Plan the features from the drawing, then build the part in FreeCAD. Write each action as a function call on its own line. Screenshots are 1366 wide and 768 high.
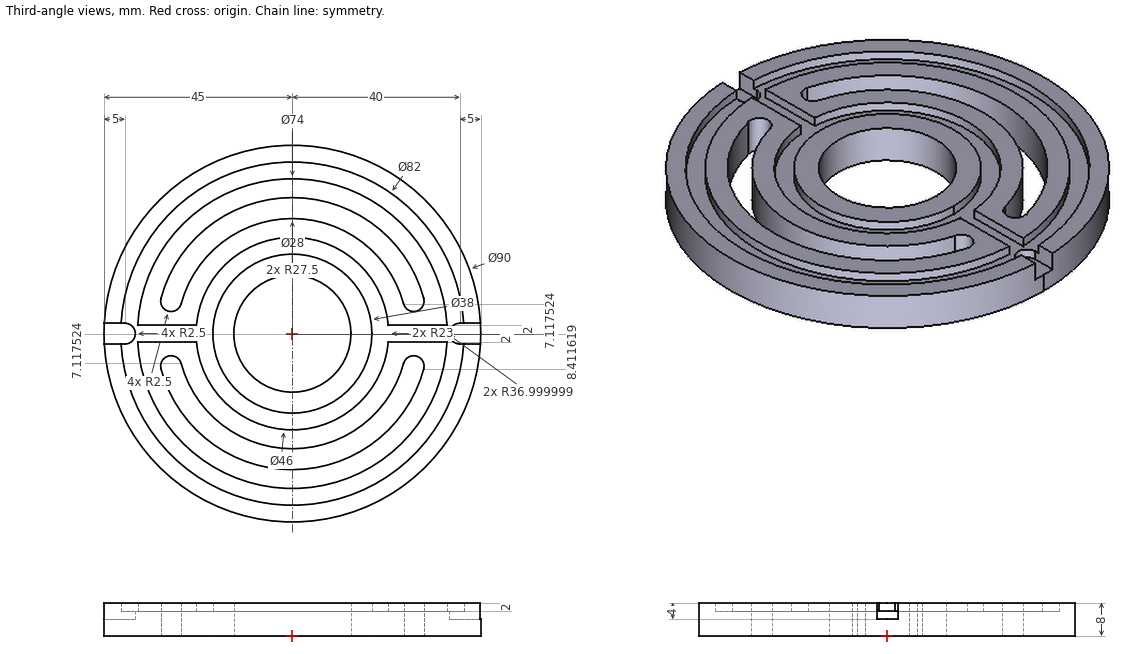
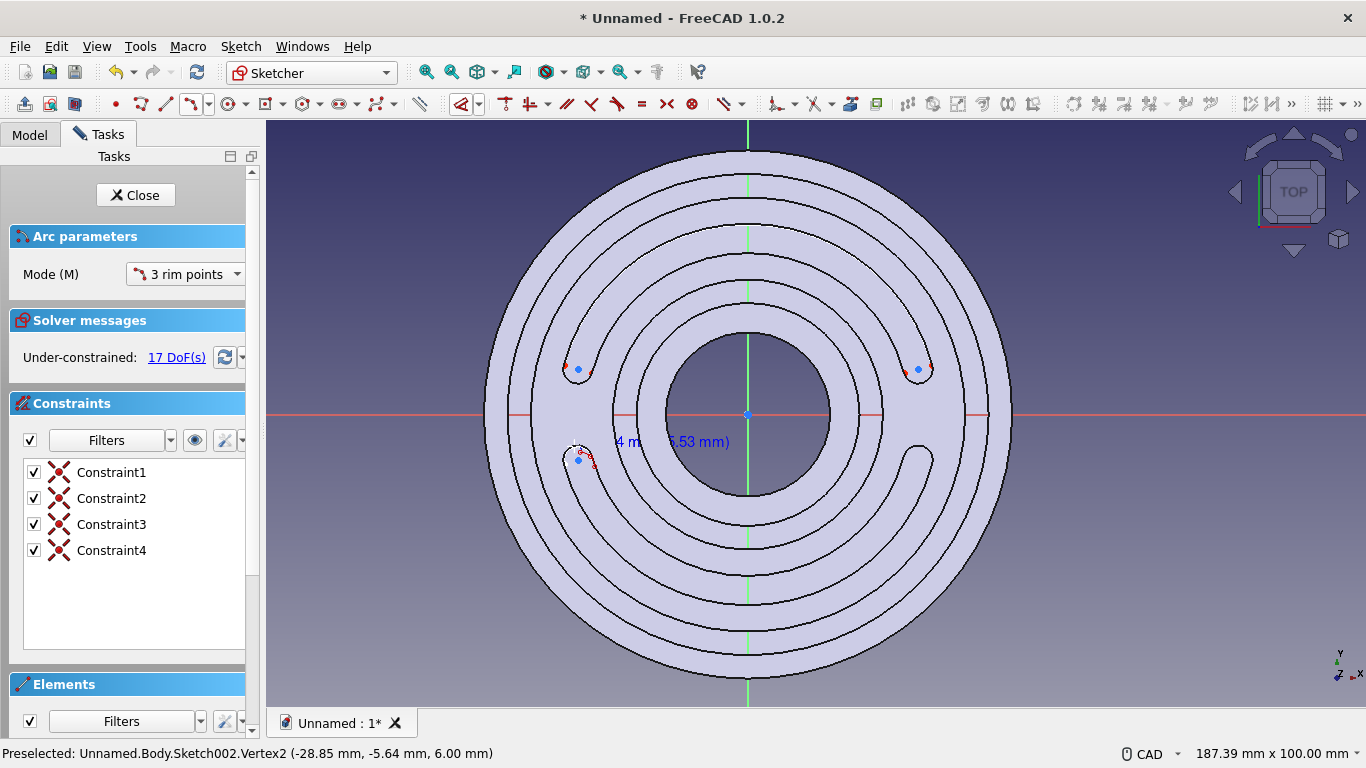
click(564, 465)
click(932, 464)
click(699, 599)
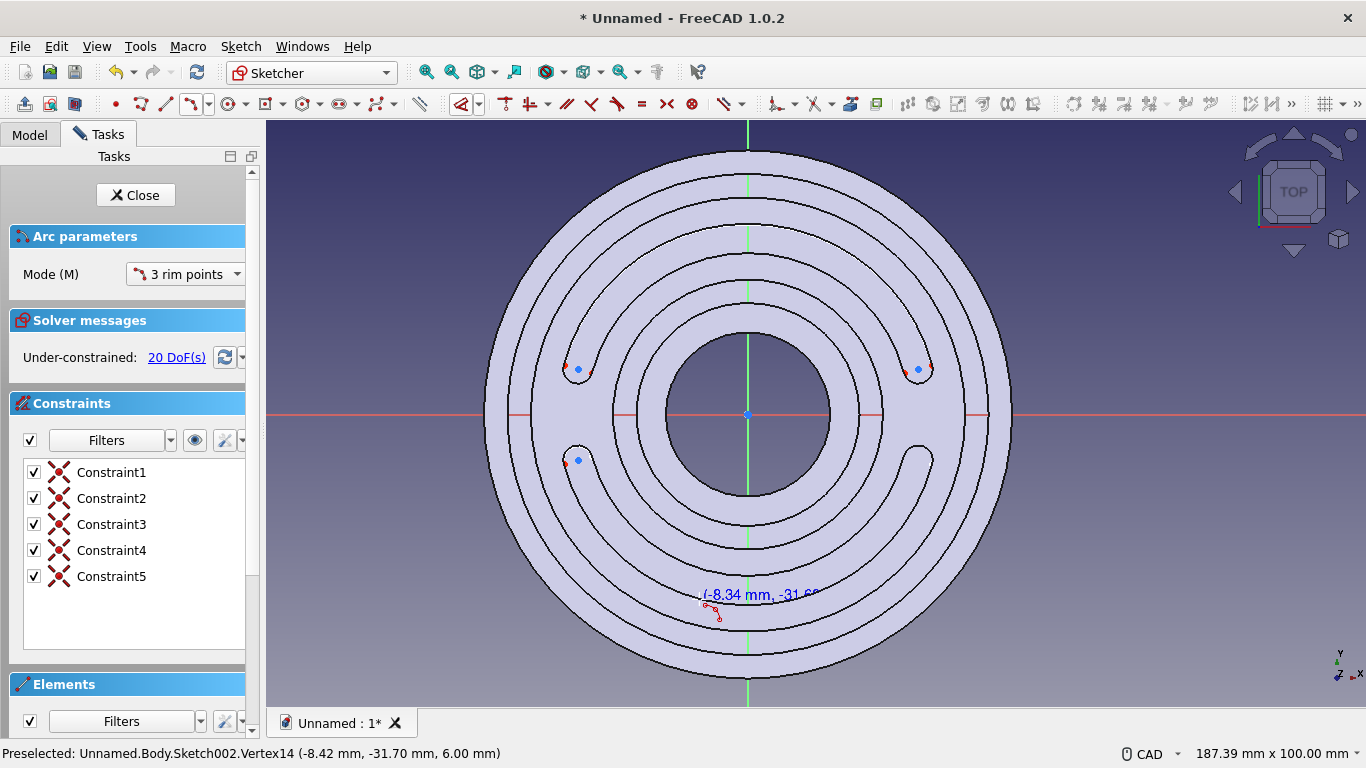
click(932, 465)
click(904, 456)
click(922, 446)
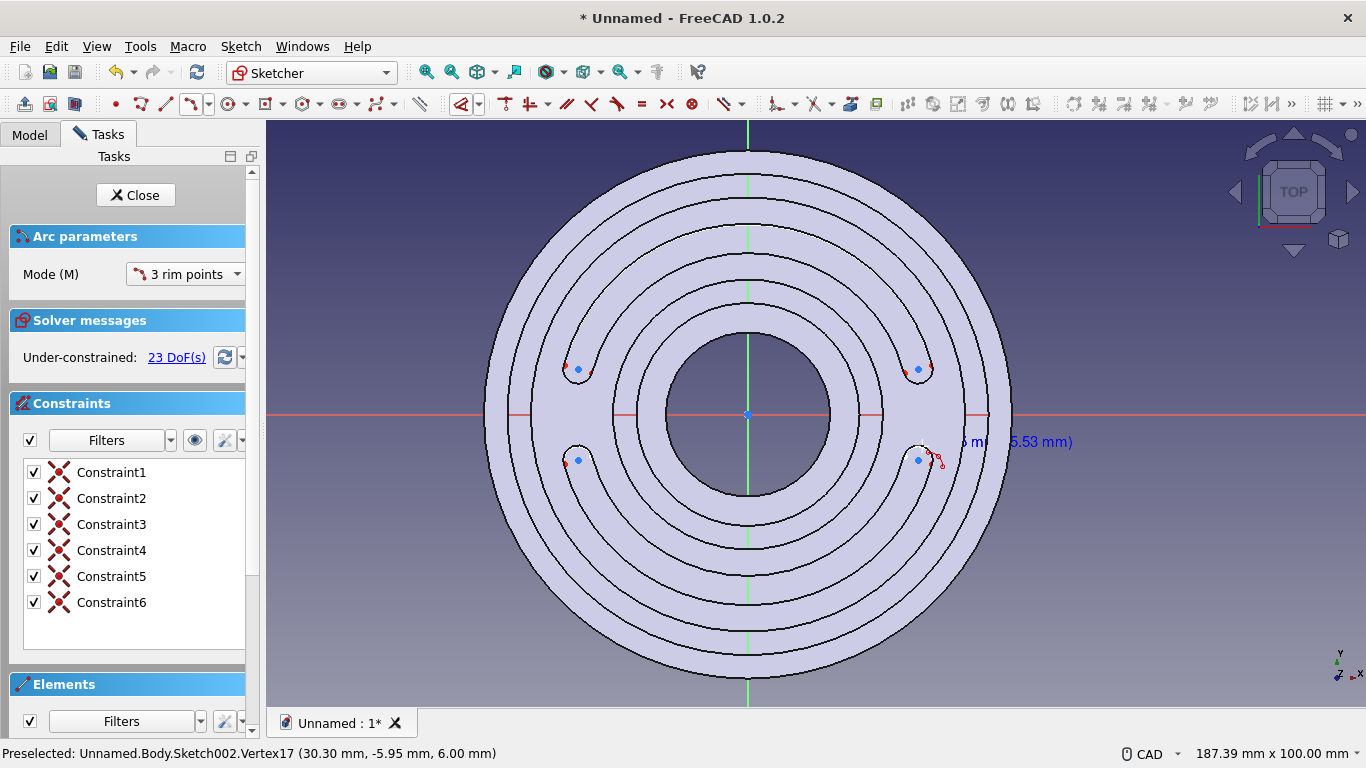
click(904, 457)
click(592, 457)
click(706, 570)
key(Escape)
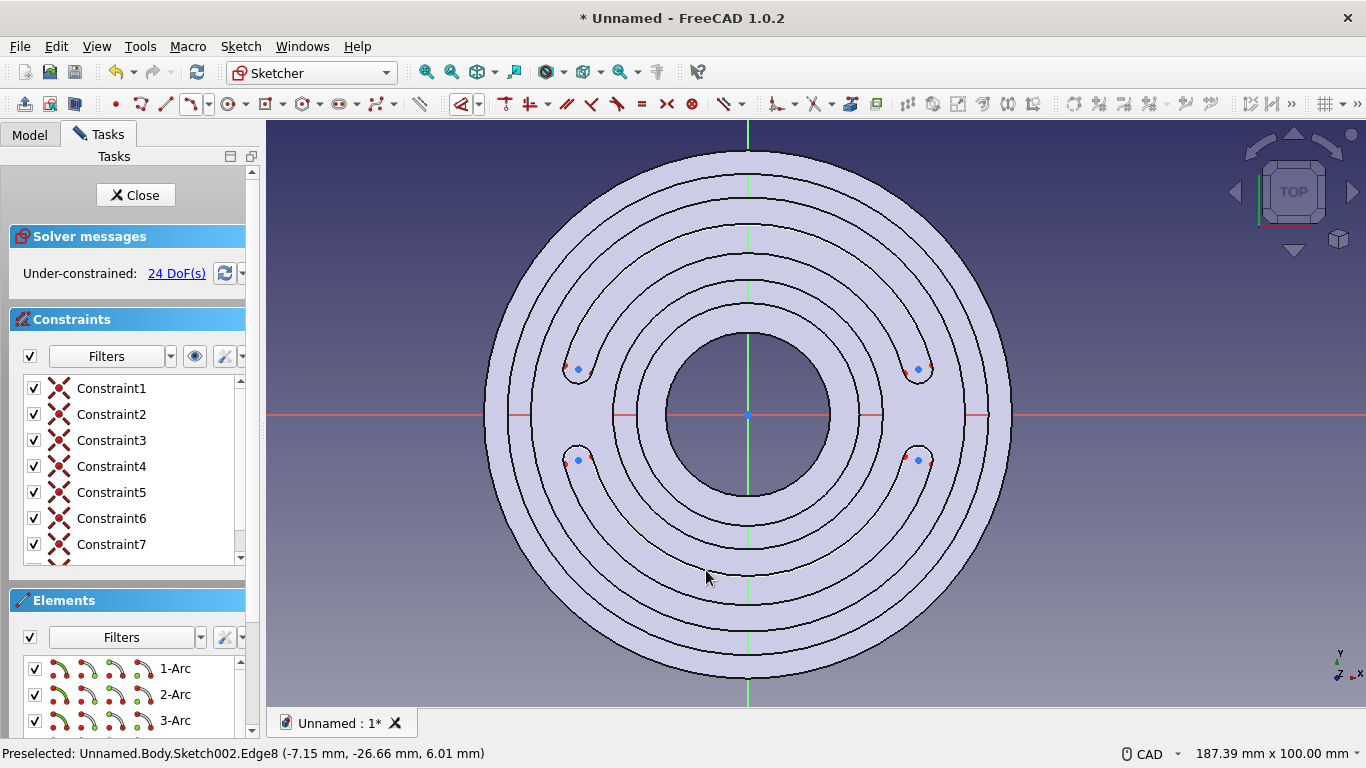
click(829, 276)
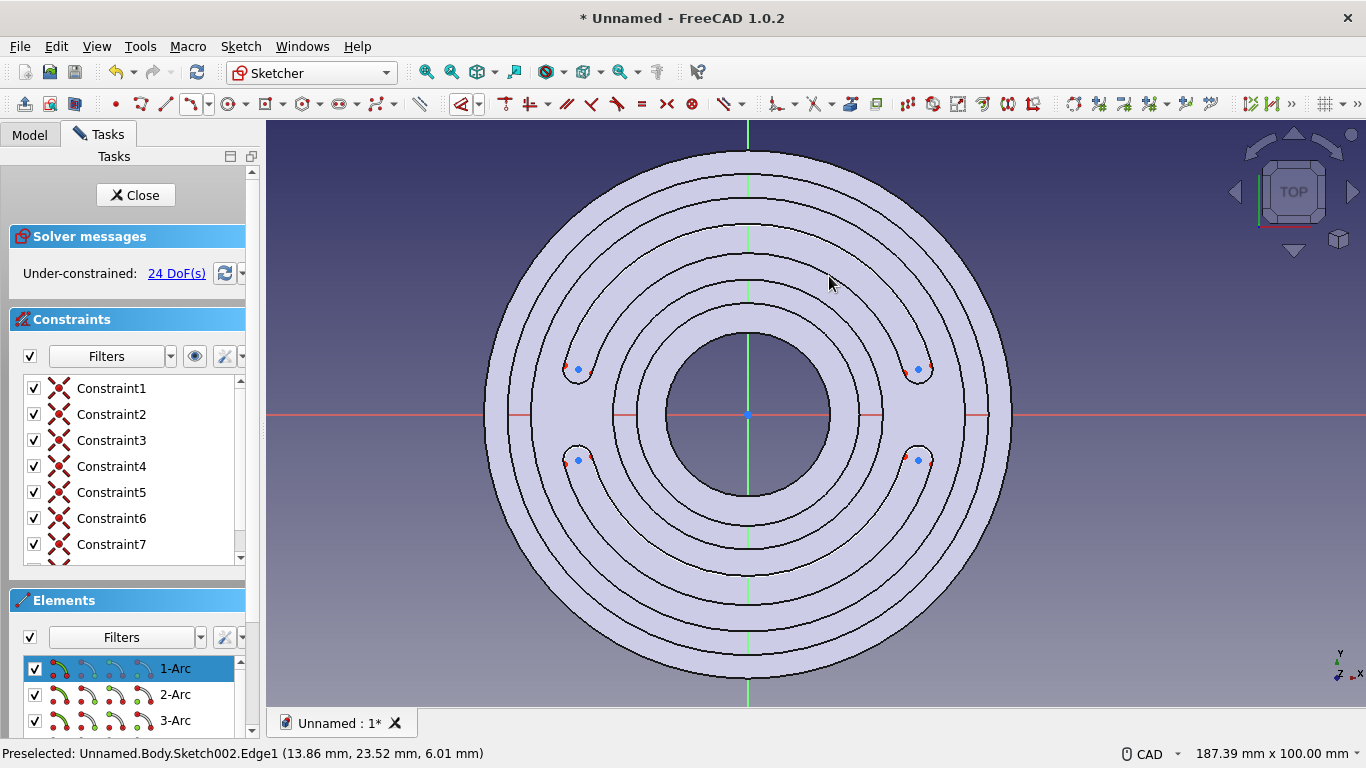
click(913, 384)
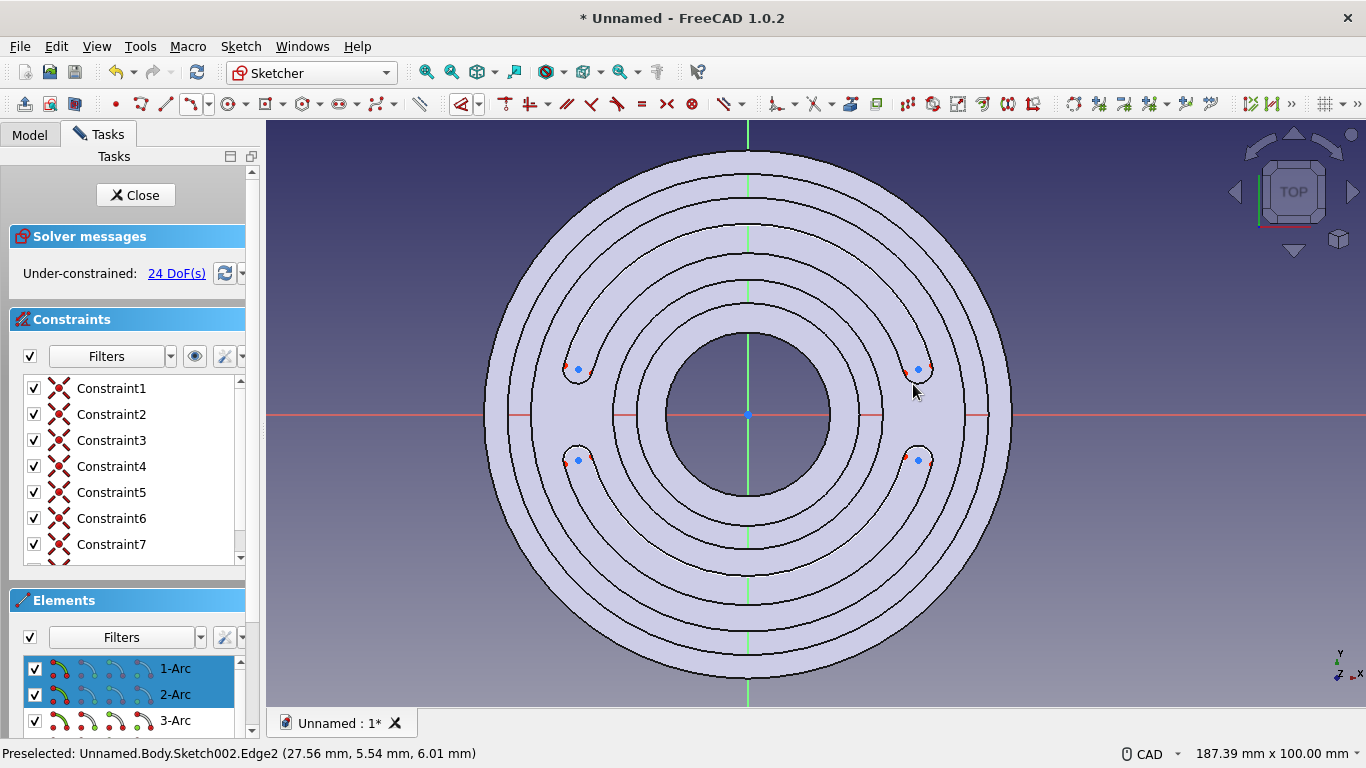
key(t)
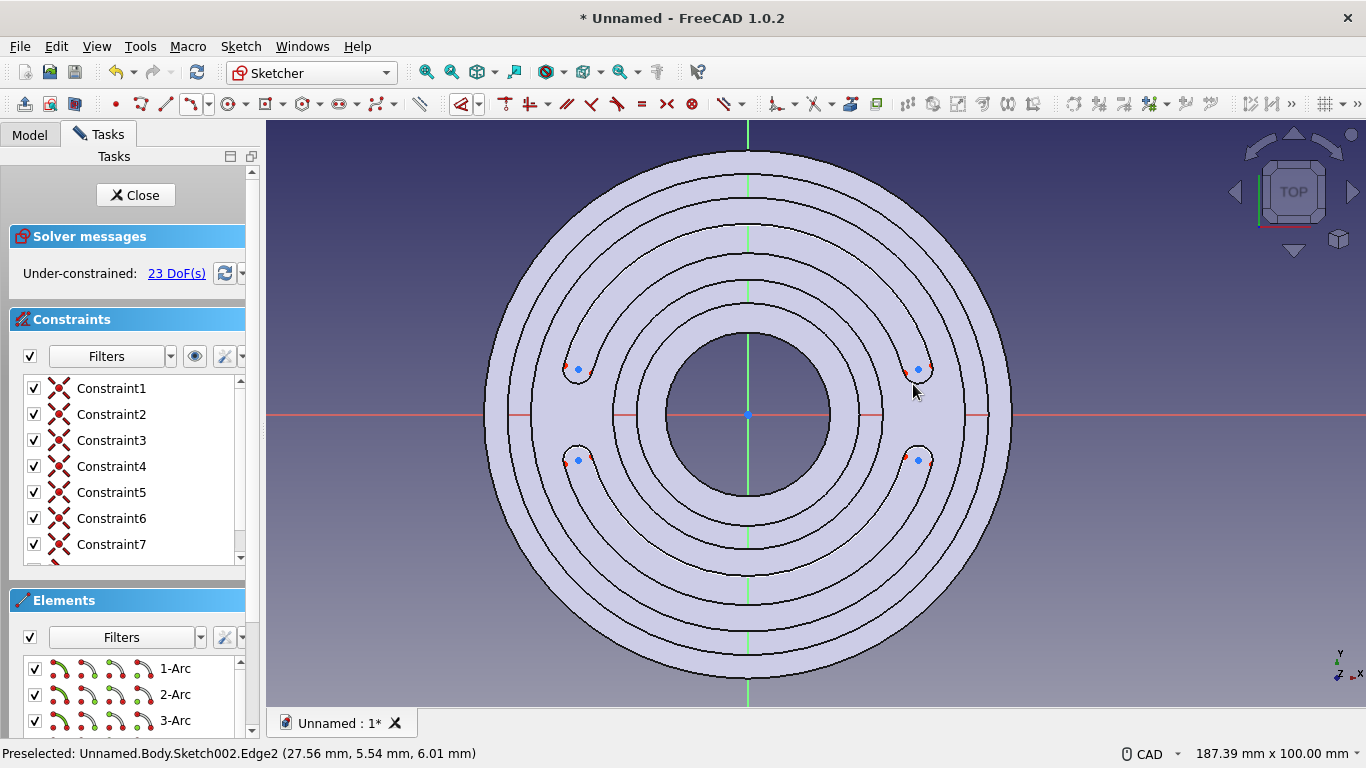
click(829, 276)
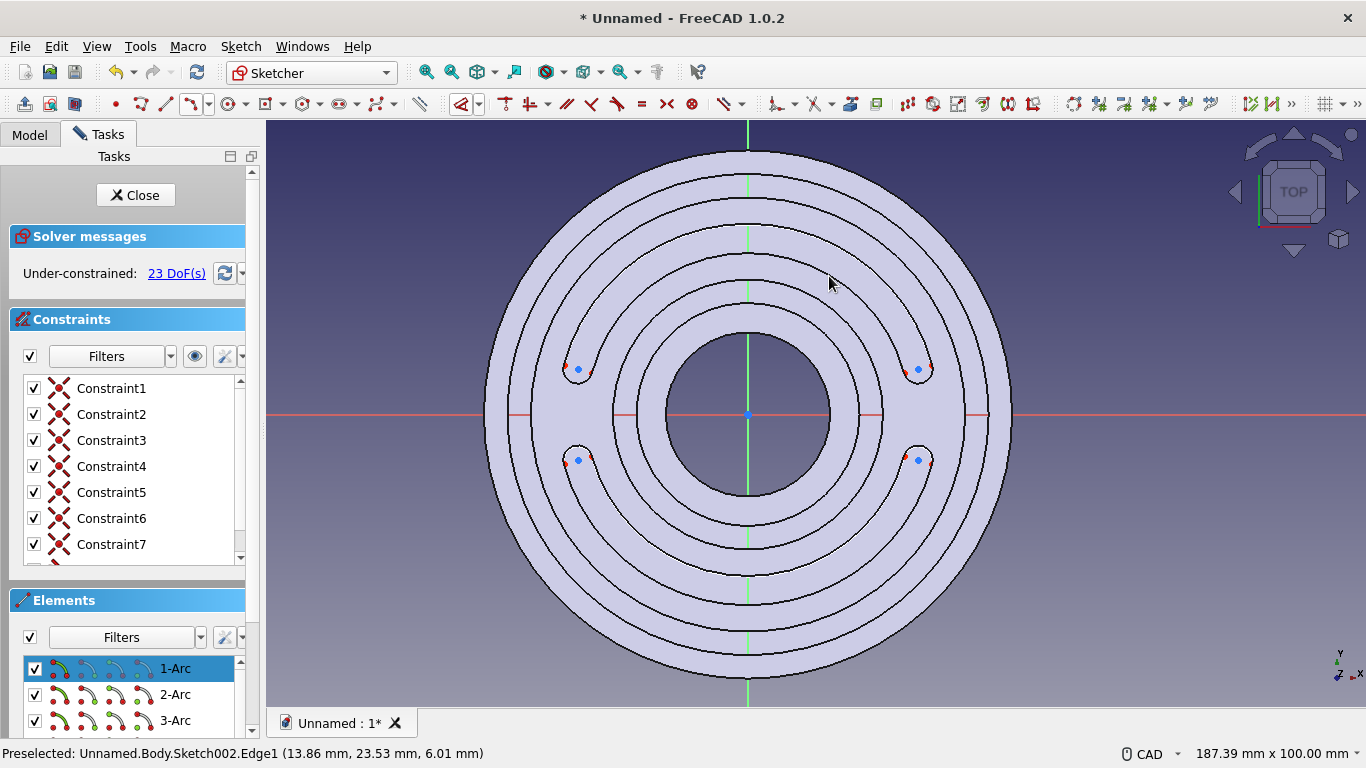
click(567, 379)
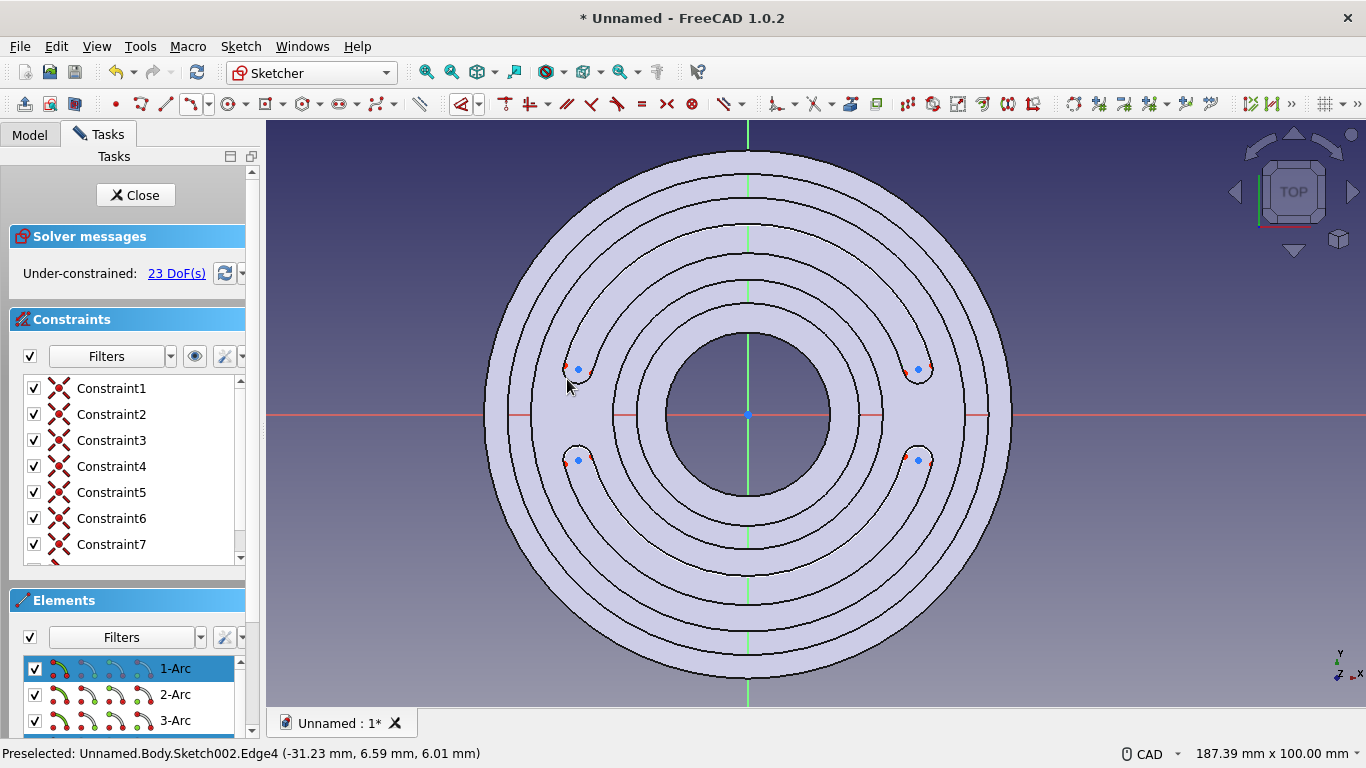
key(t)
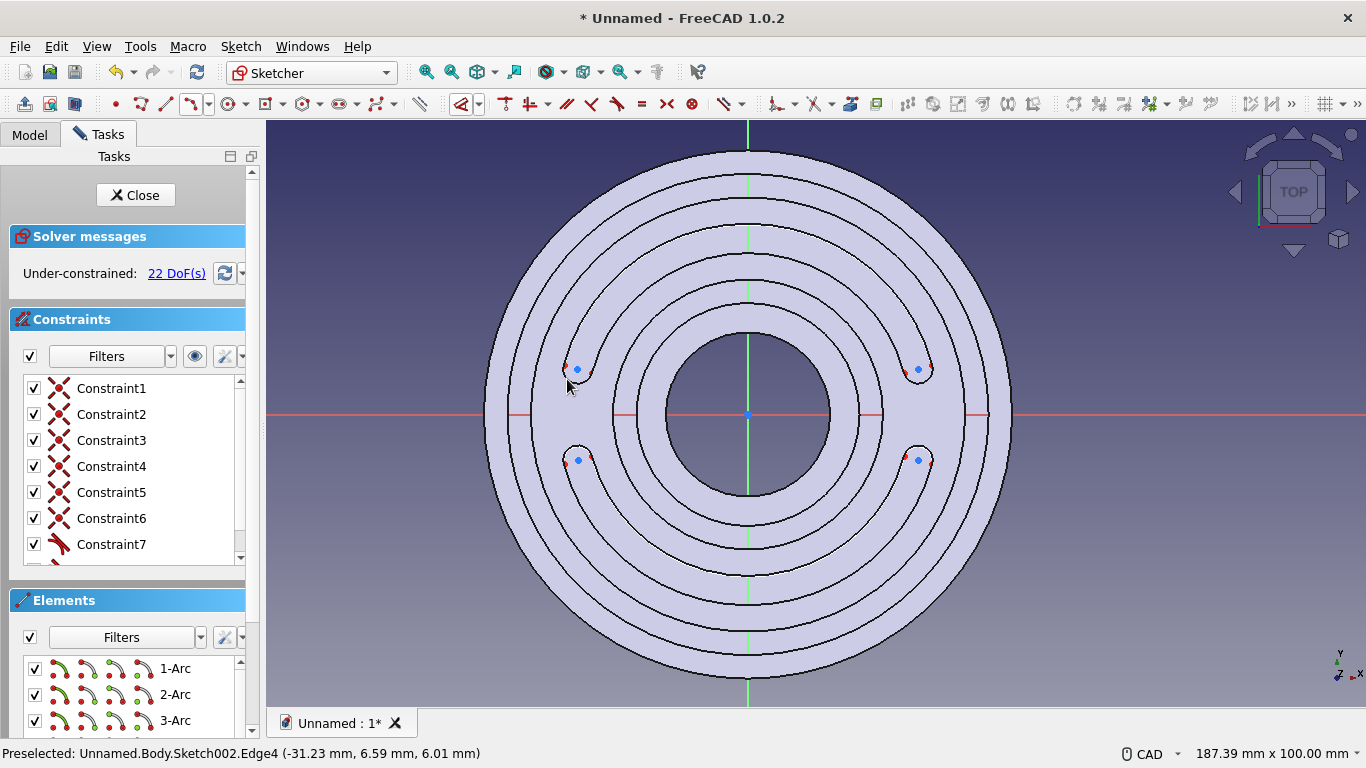
click(913, 384)